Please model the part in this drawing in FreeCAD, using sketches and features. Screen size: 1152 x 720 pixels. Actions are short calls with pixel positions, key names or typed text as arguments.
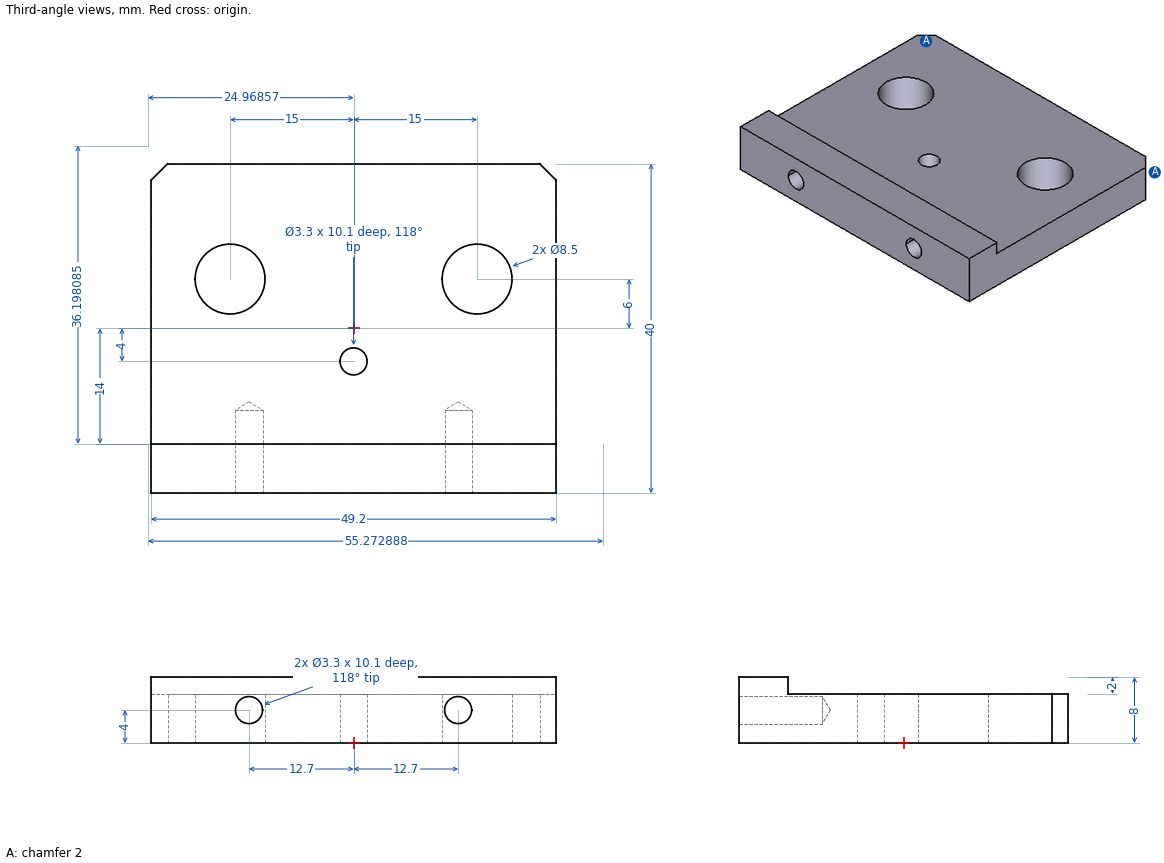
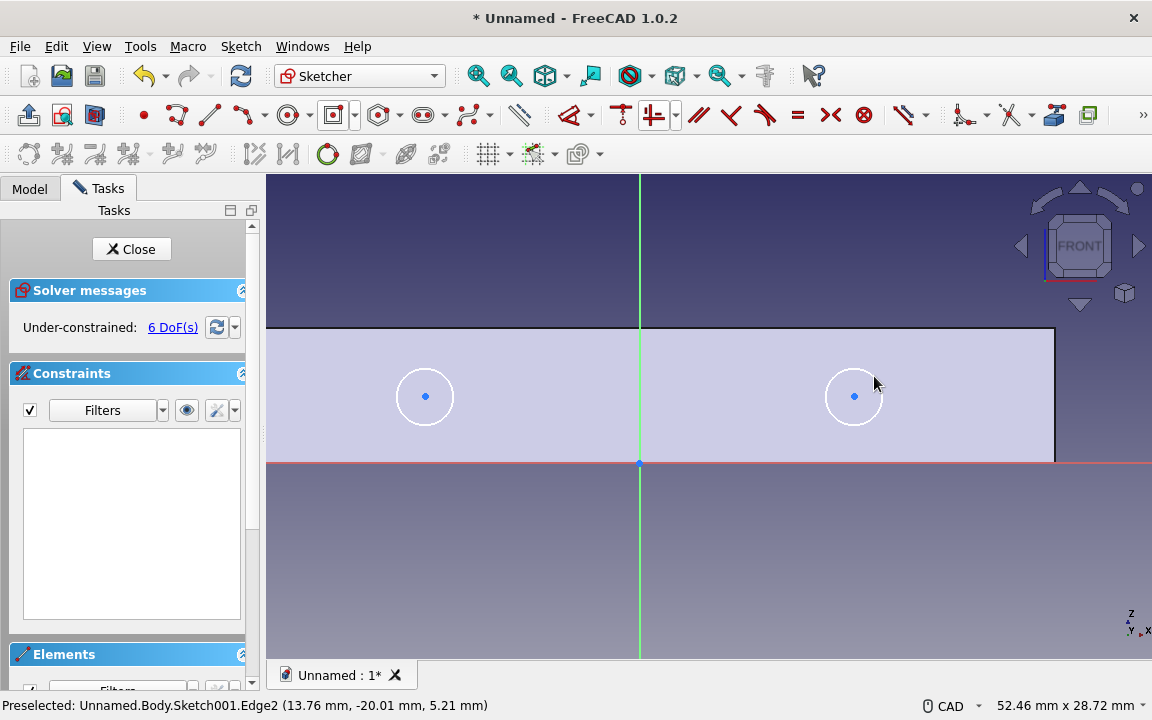
click(445, 377)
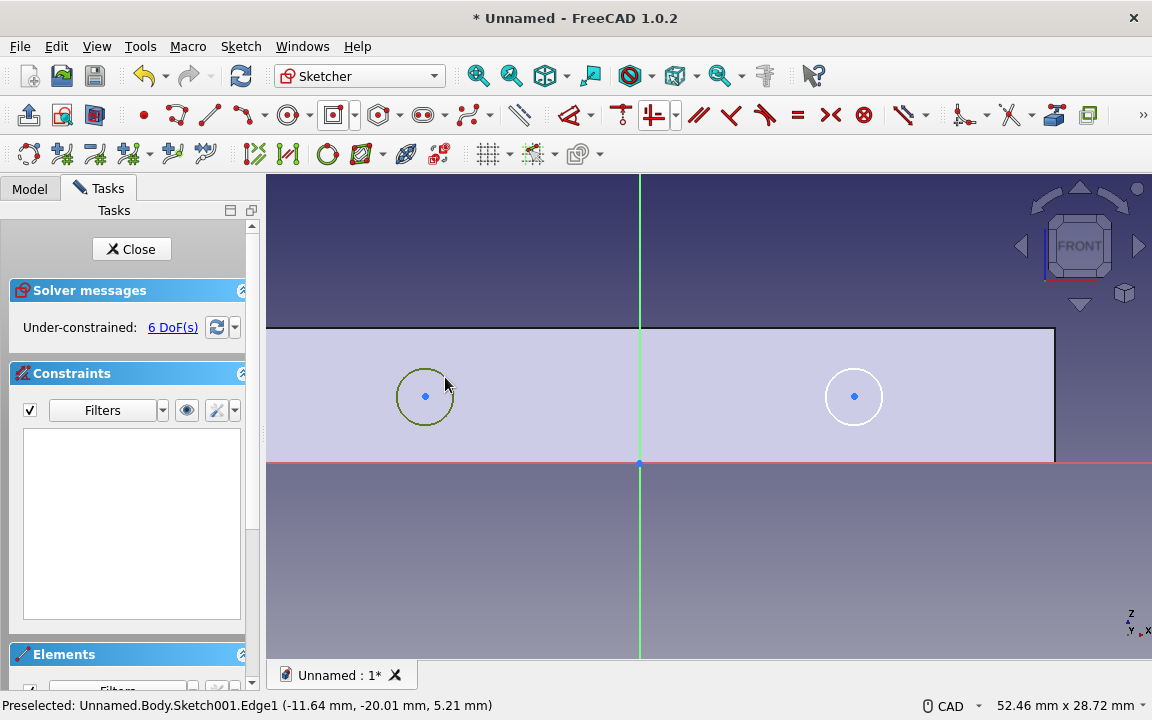
click(874, 377)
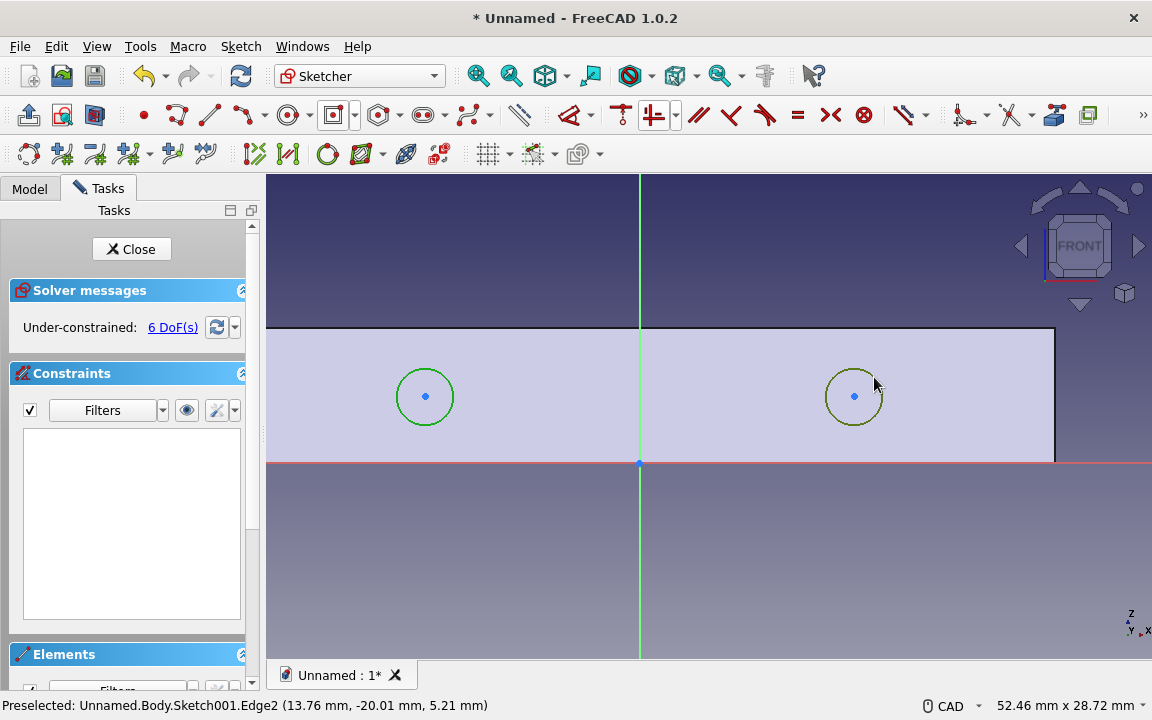
key(e)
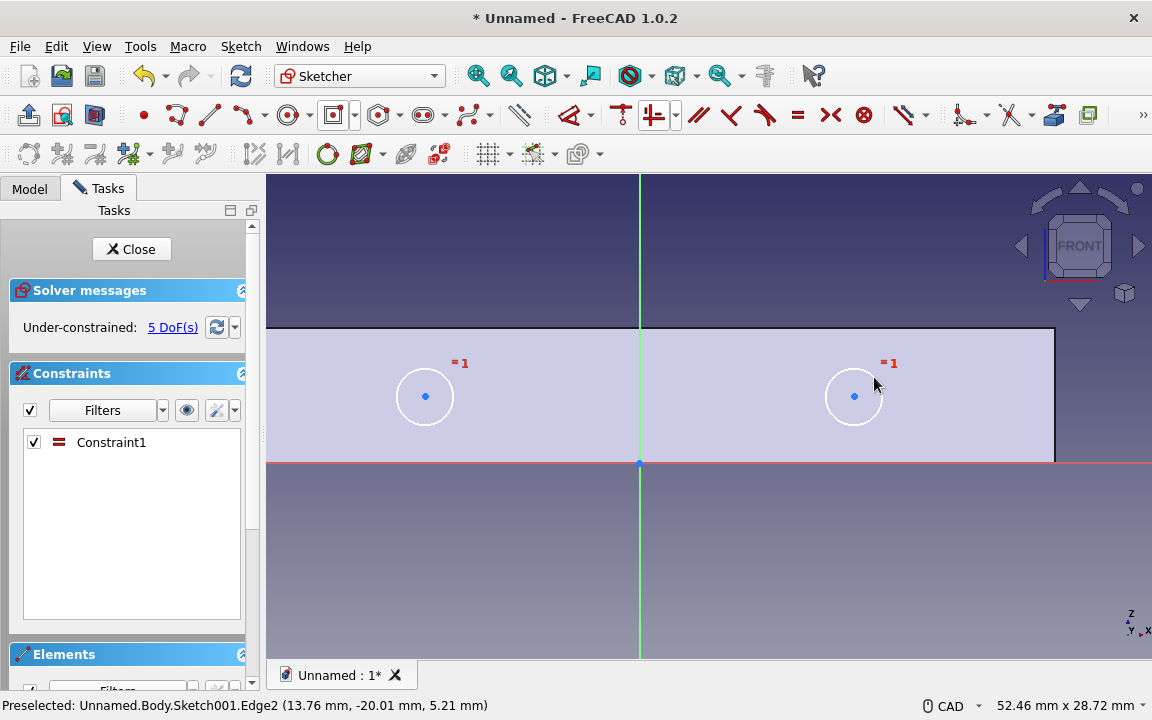
click(425, 397)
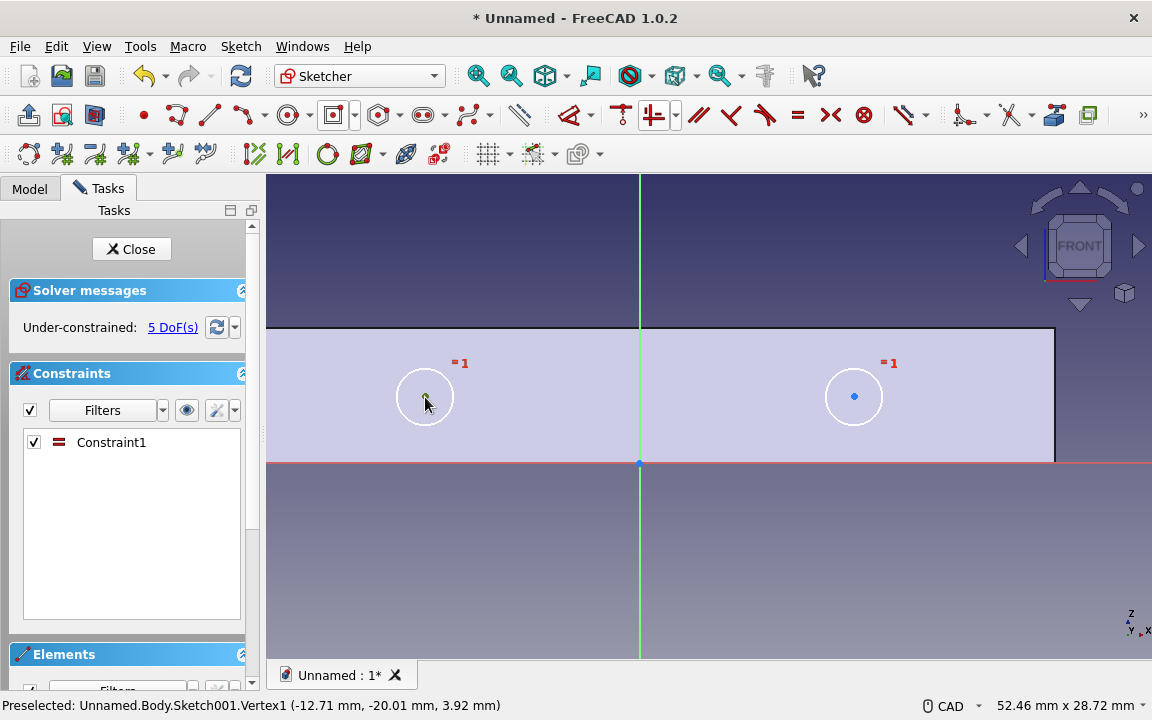
click(854, 397)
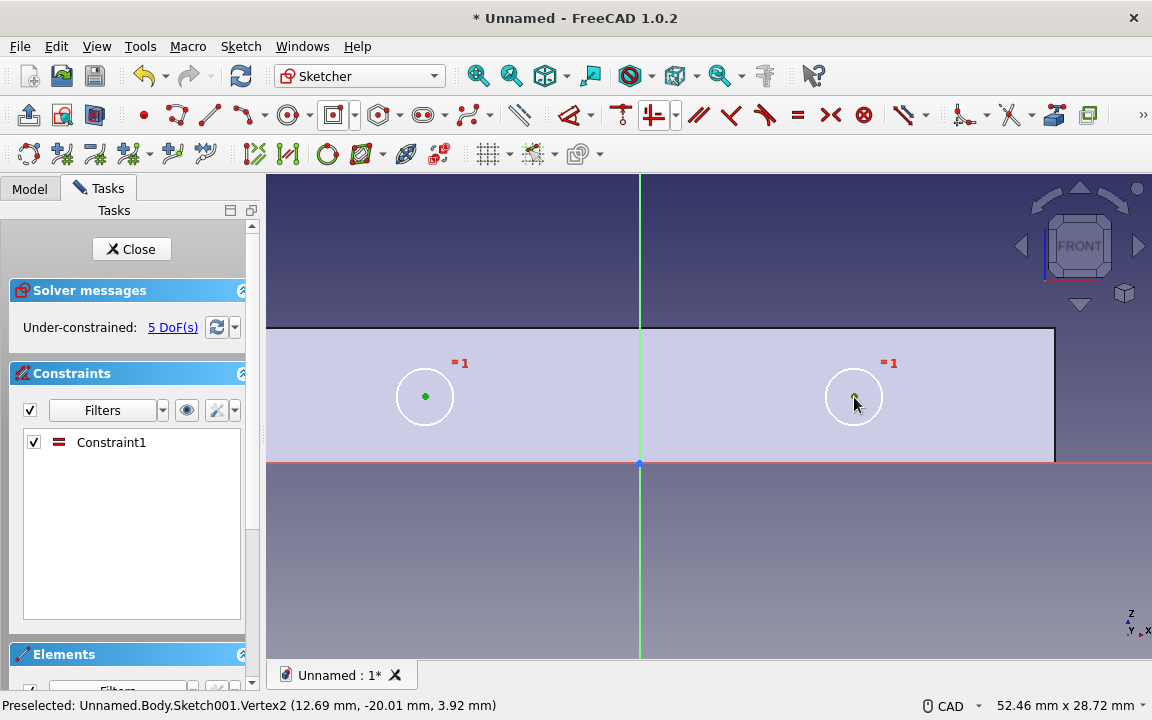
key(h)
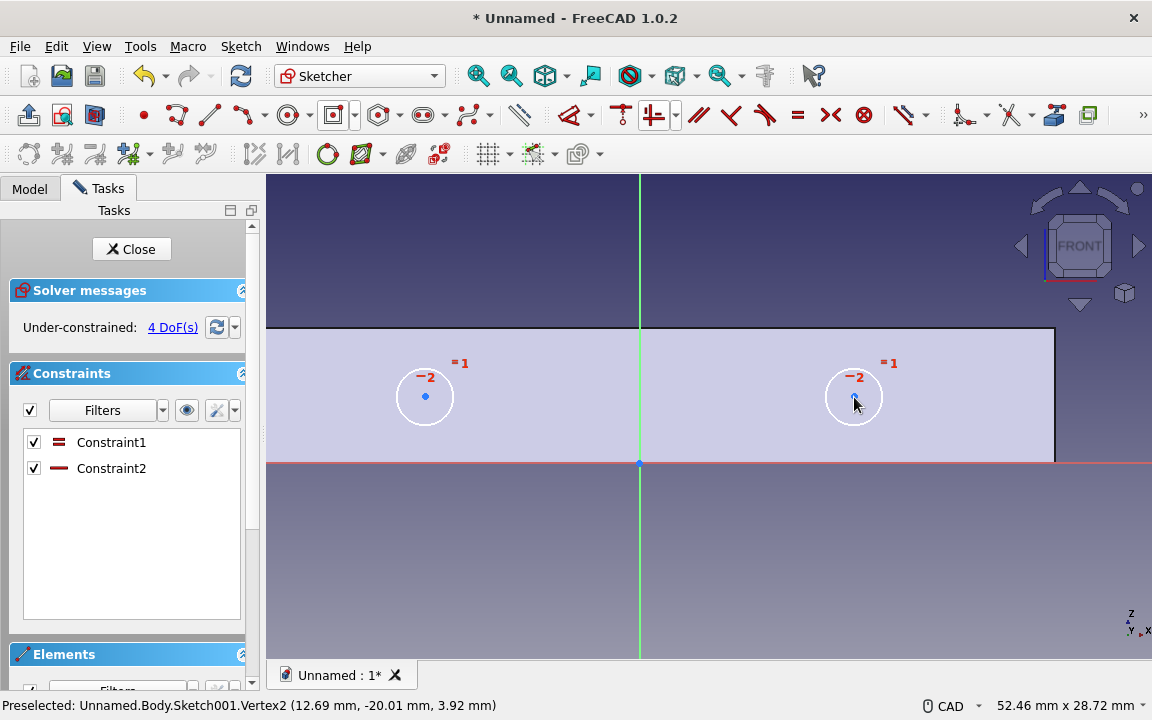
key(d)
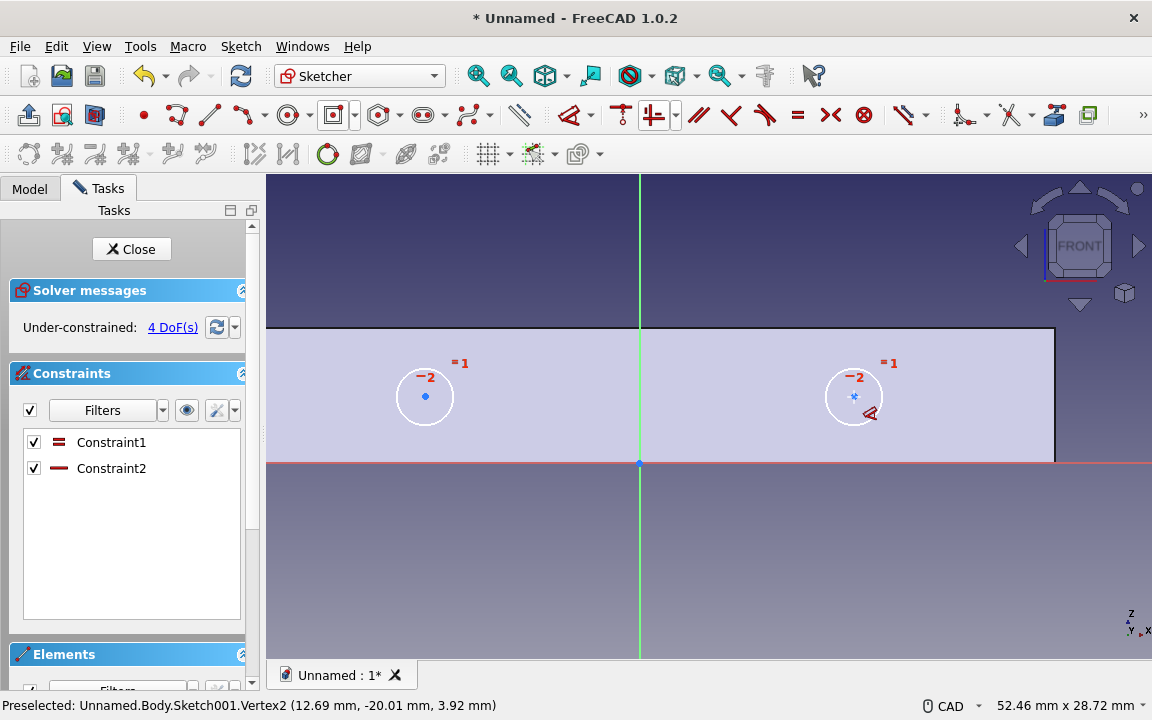
click(445, 377)
click(468, 354)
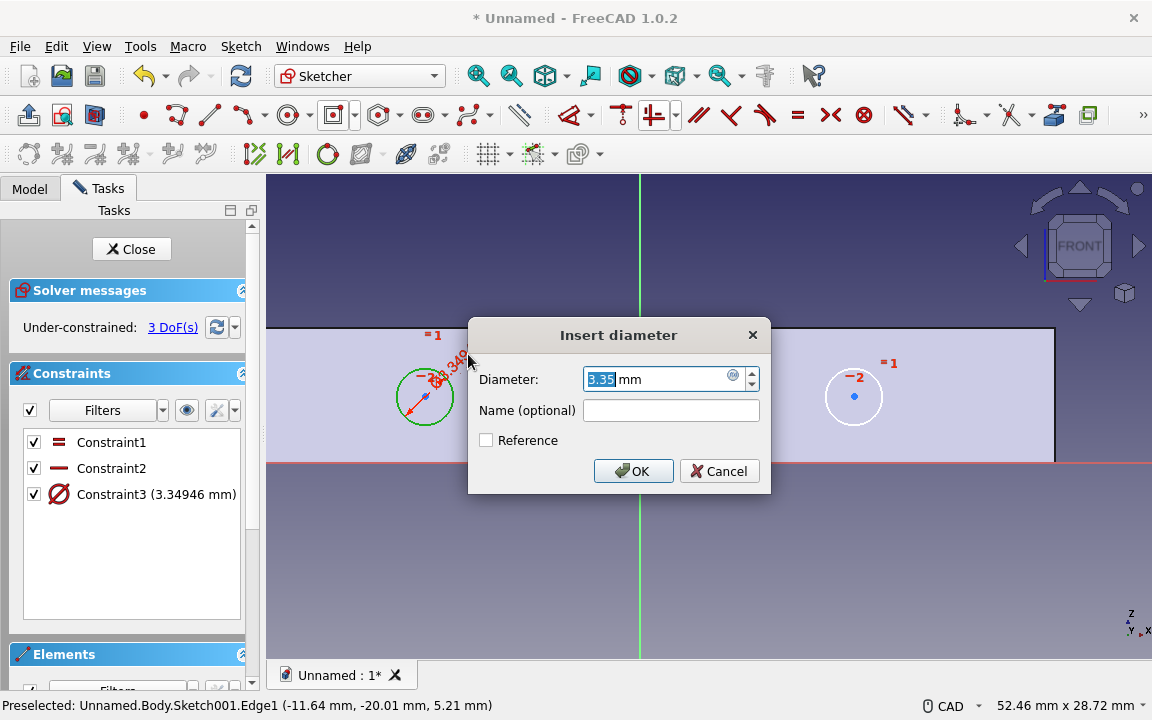
text(3.3)
key(Return)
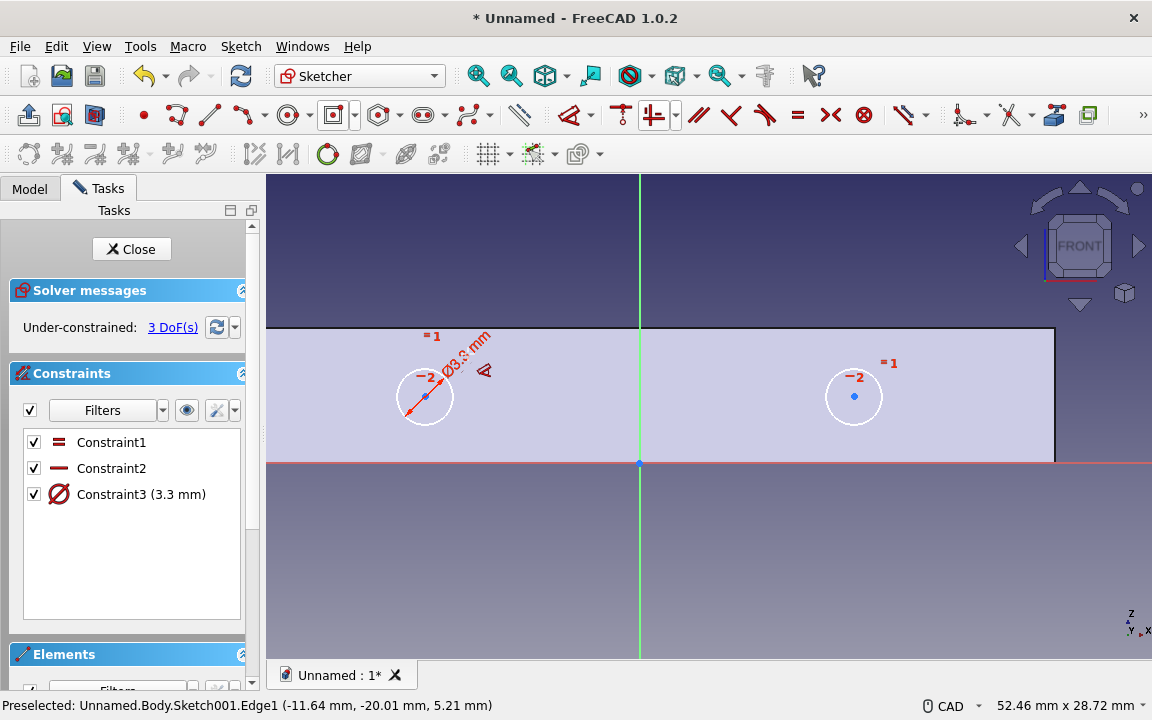
click(425, 397)
click(391, 430)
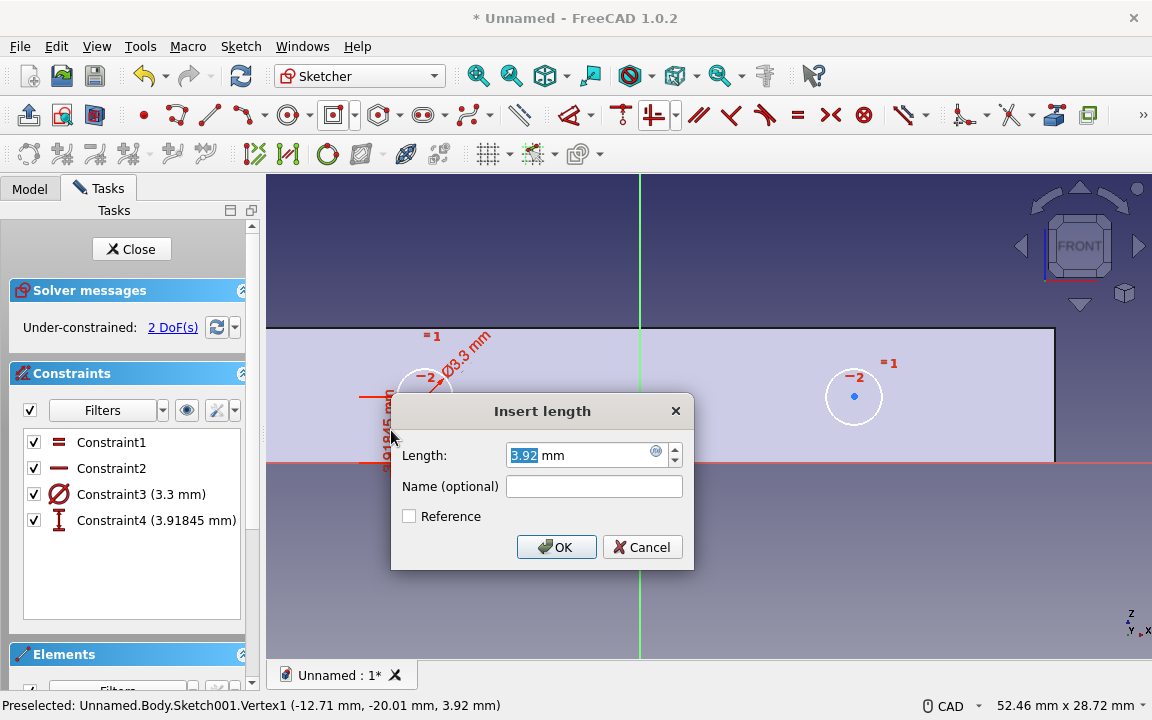
text(4)
key(Return)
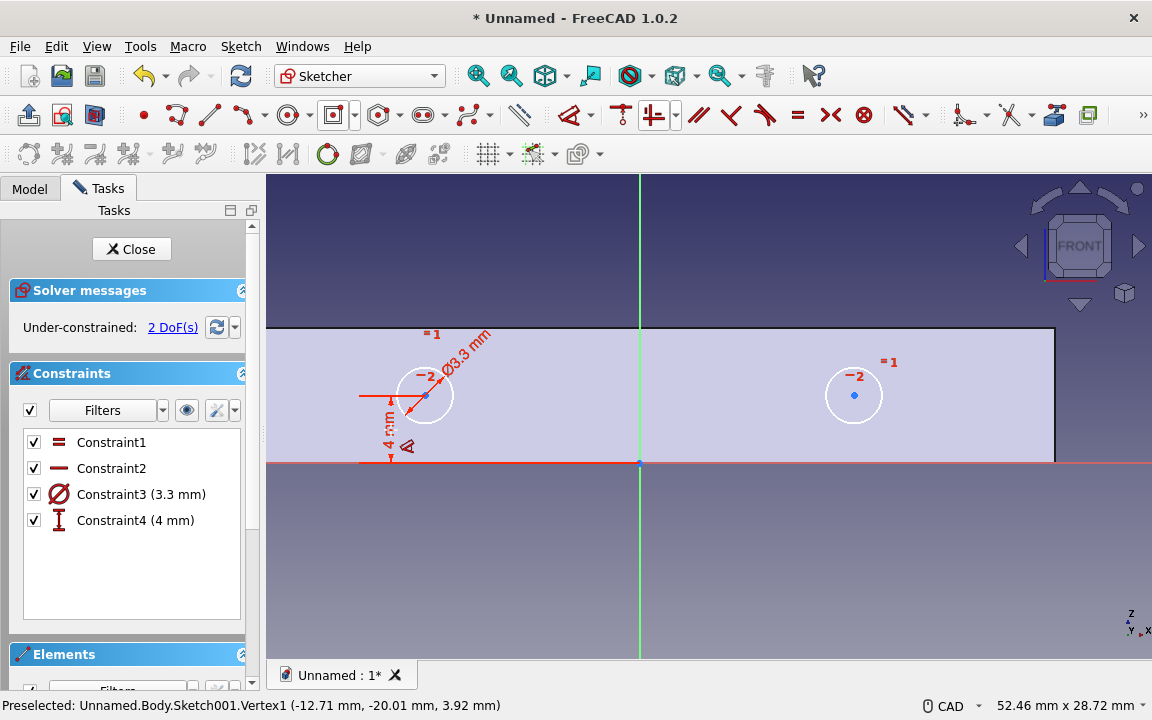
click(425, 396)
click(532, 497)